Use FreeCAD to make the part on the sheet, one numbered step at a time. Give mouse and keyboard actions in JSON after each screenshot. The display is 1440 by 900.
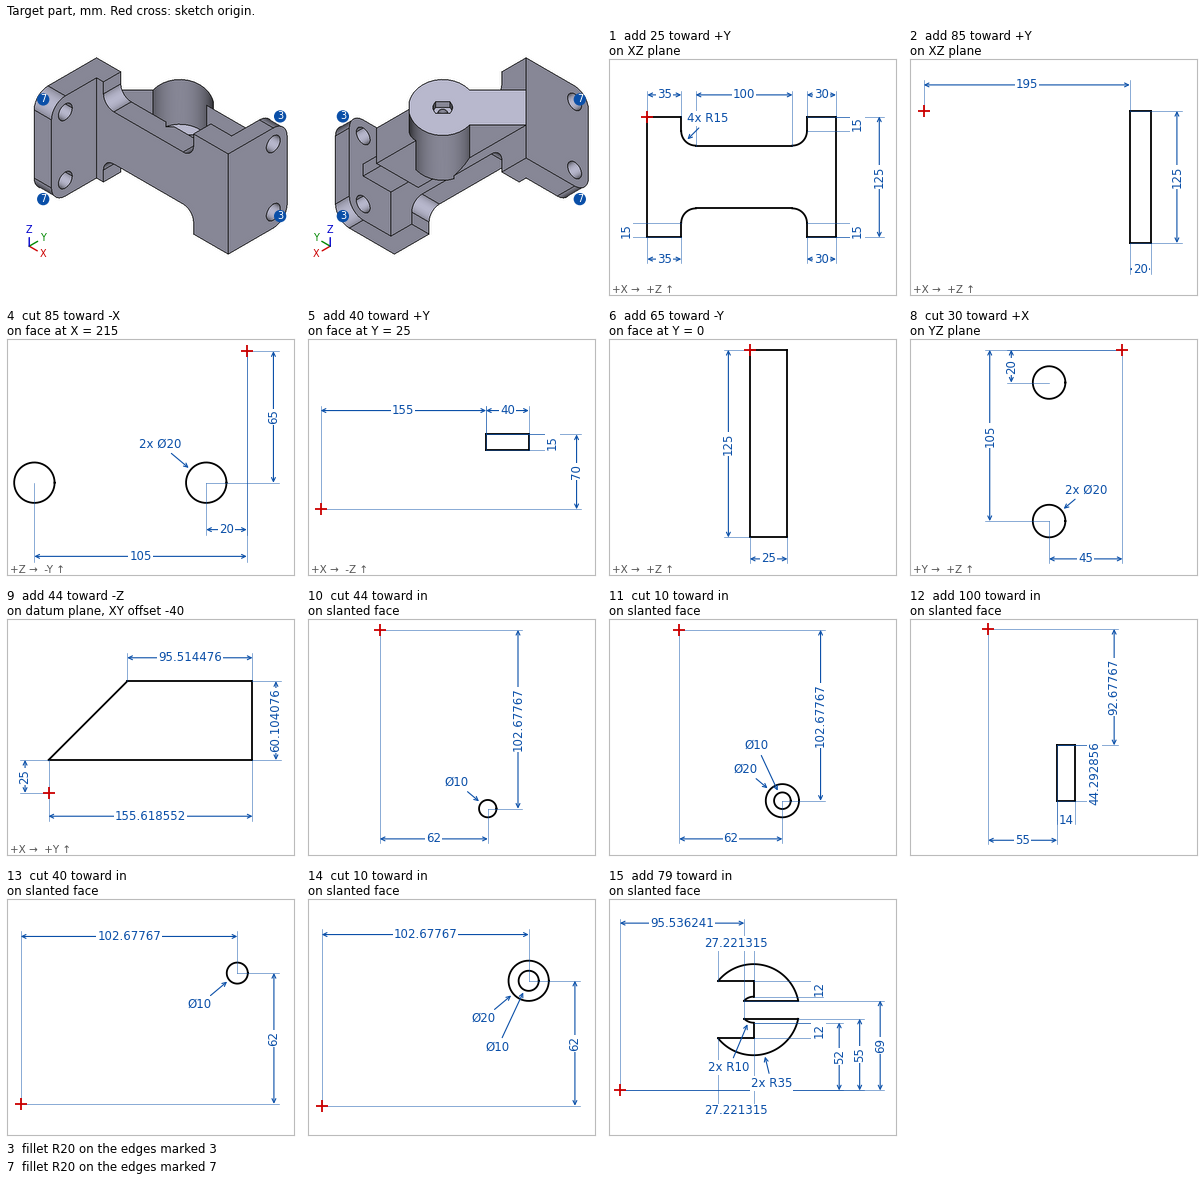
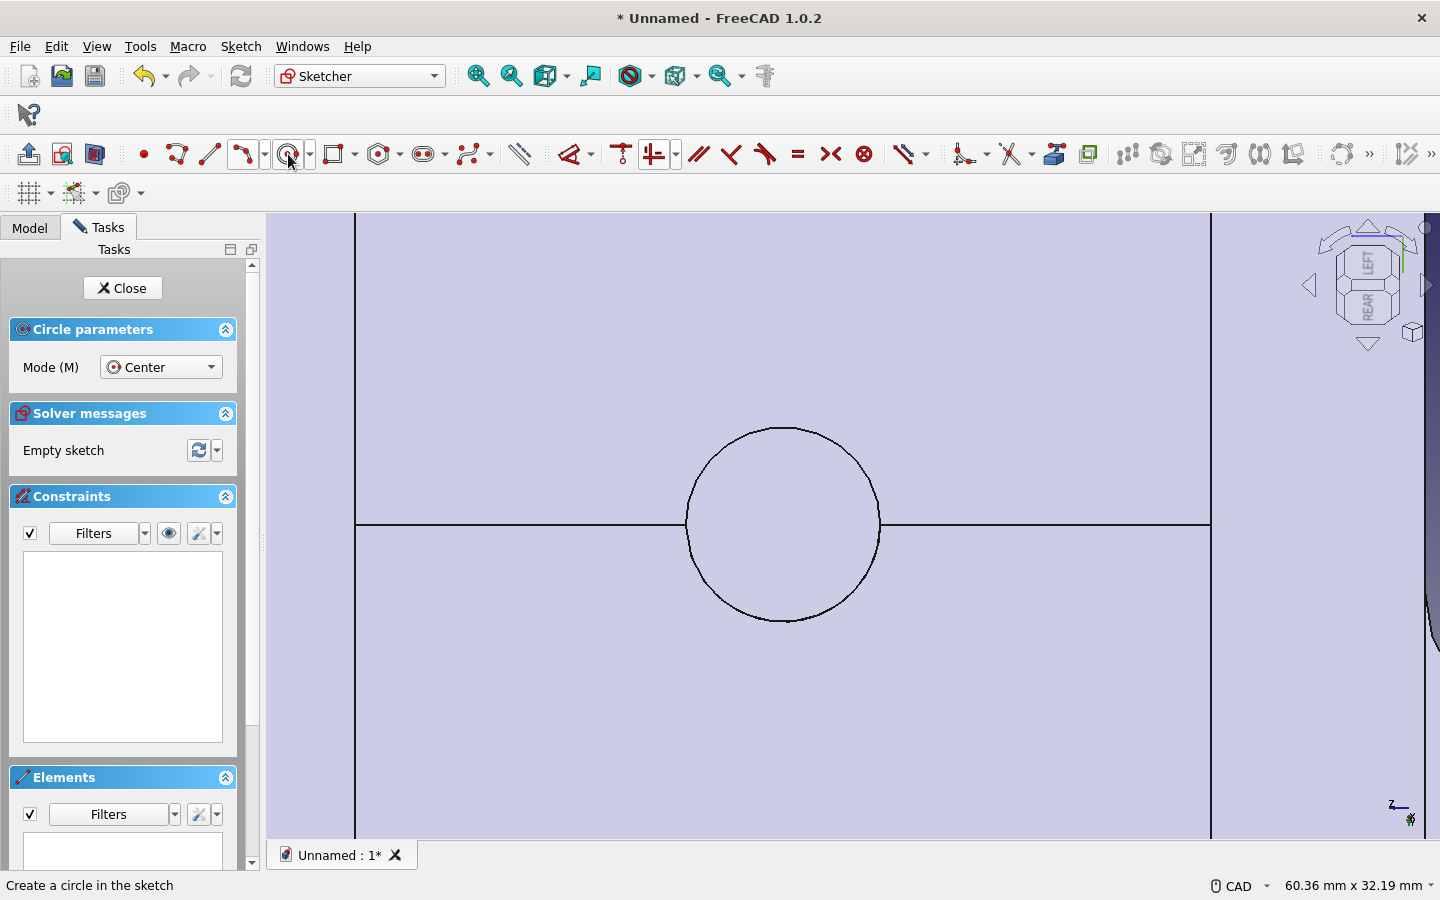
{"action": "left_click", "coordinate": [783, 525]}
{"action": "left_click", "coordinate": [921, 387]}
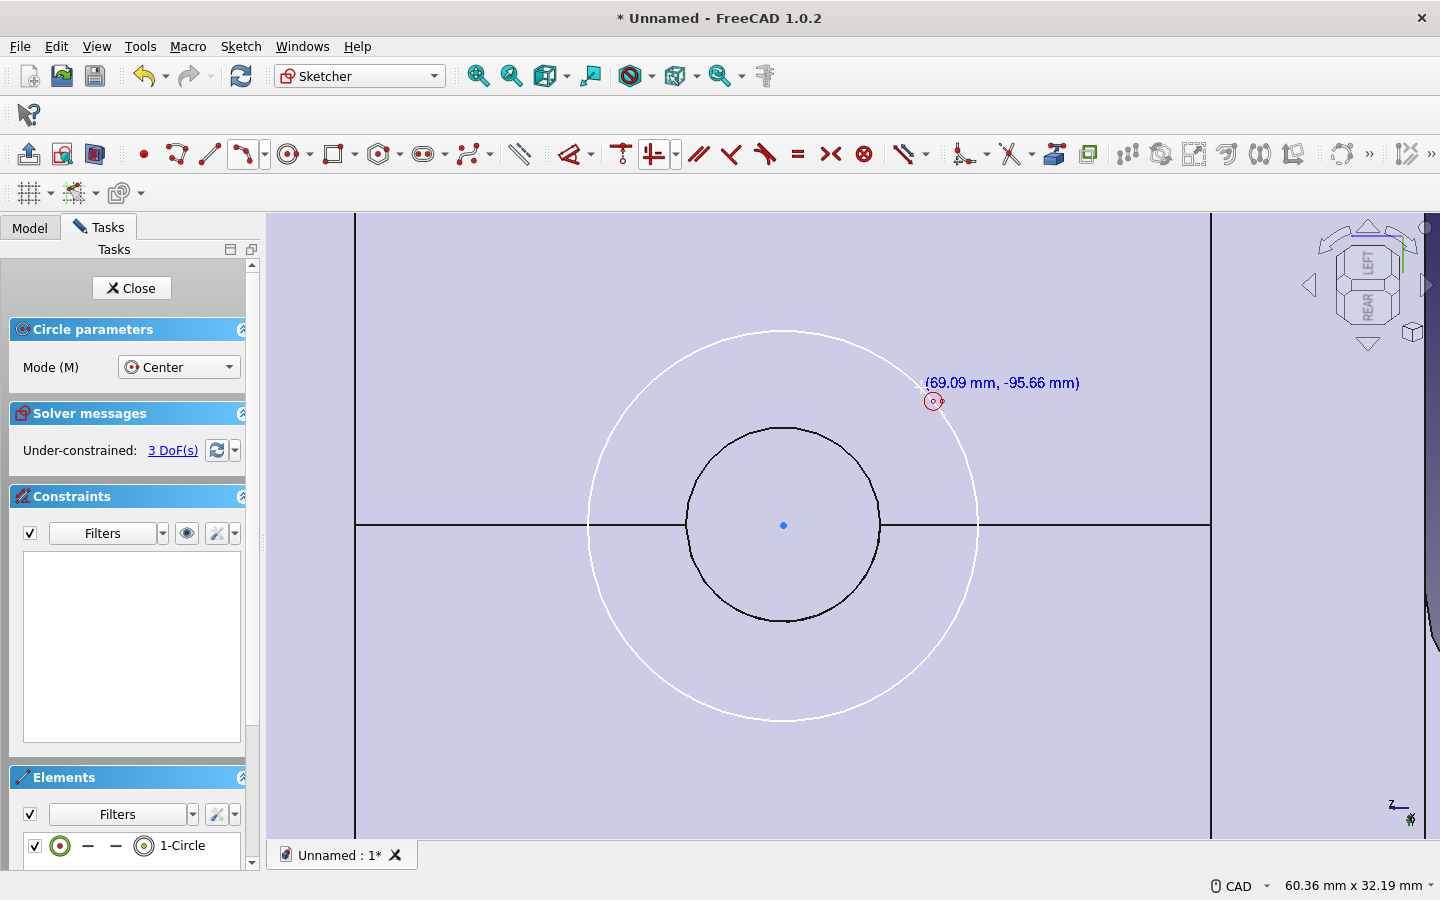
{"action": "left_click", "coordinate": [783, 526]}
{"action": "left_click", "coordinate": [852, 456]}
{"action": "key", "text": "Escape"}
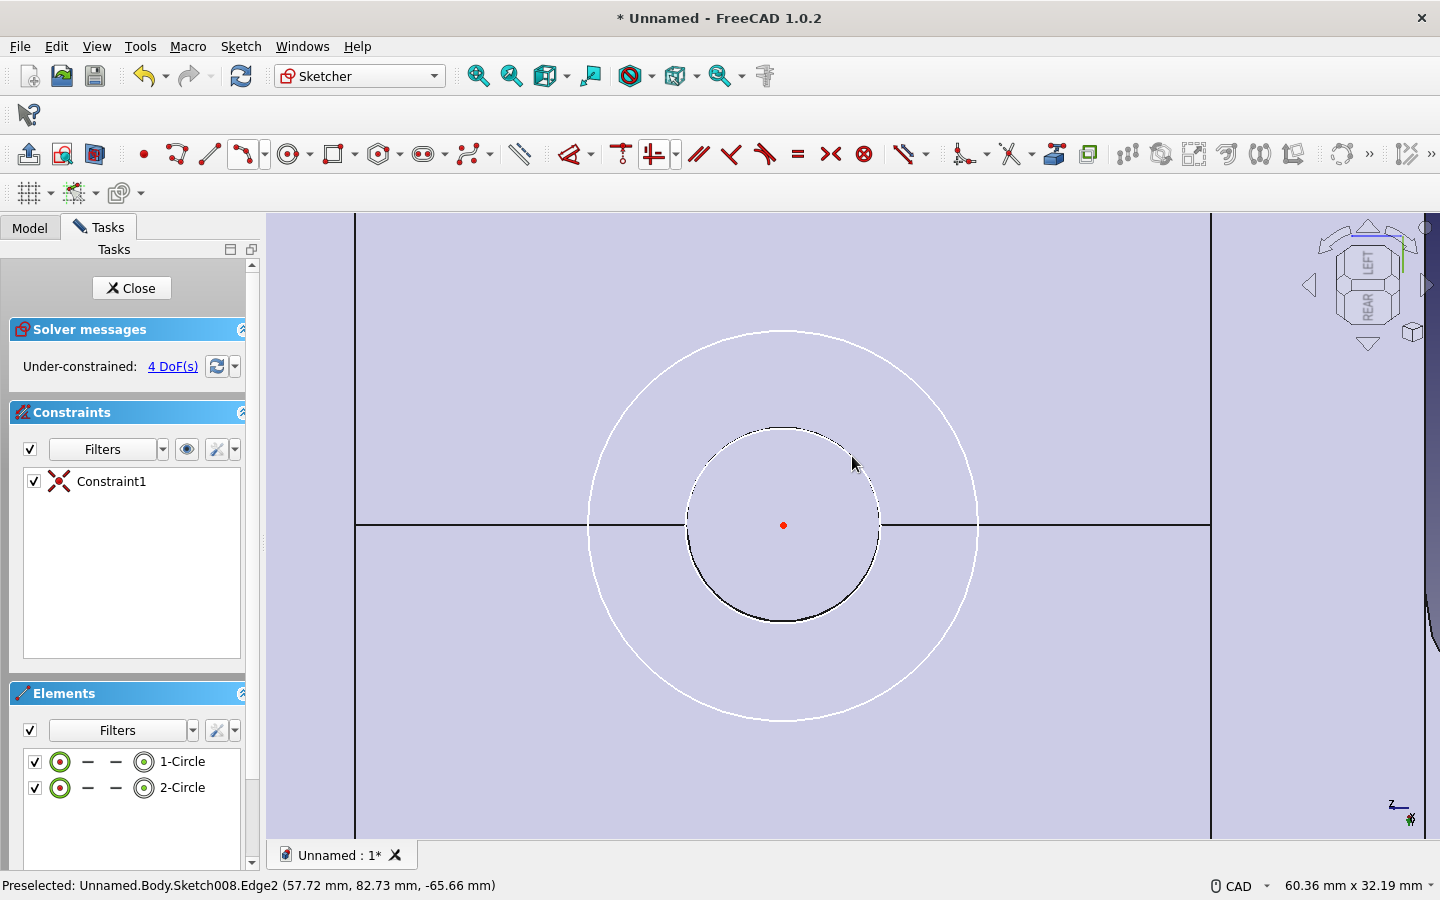
{"action": "left_click", "coordinate": [568, 154]}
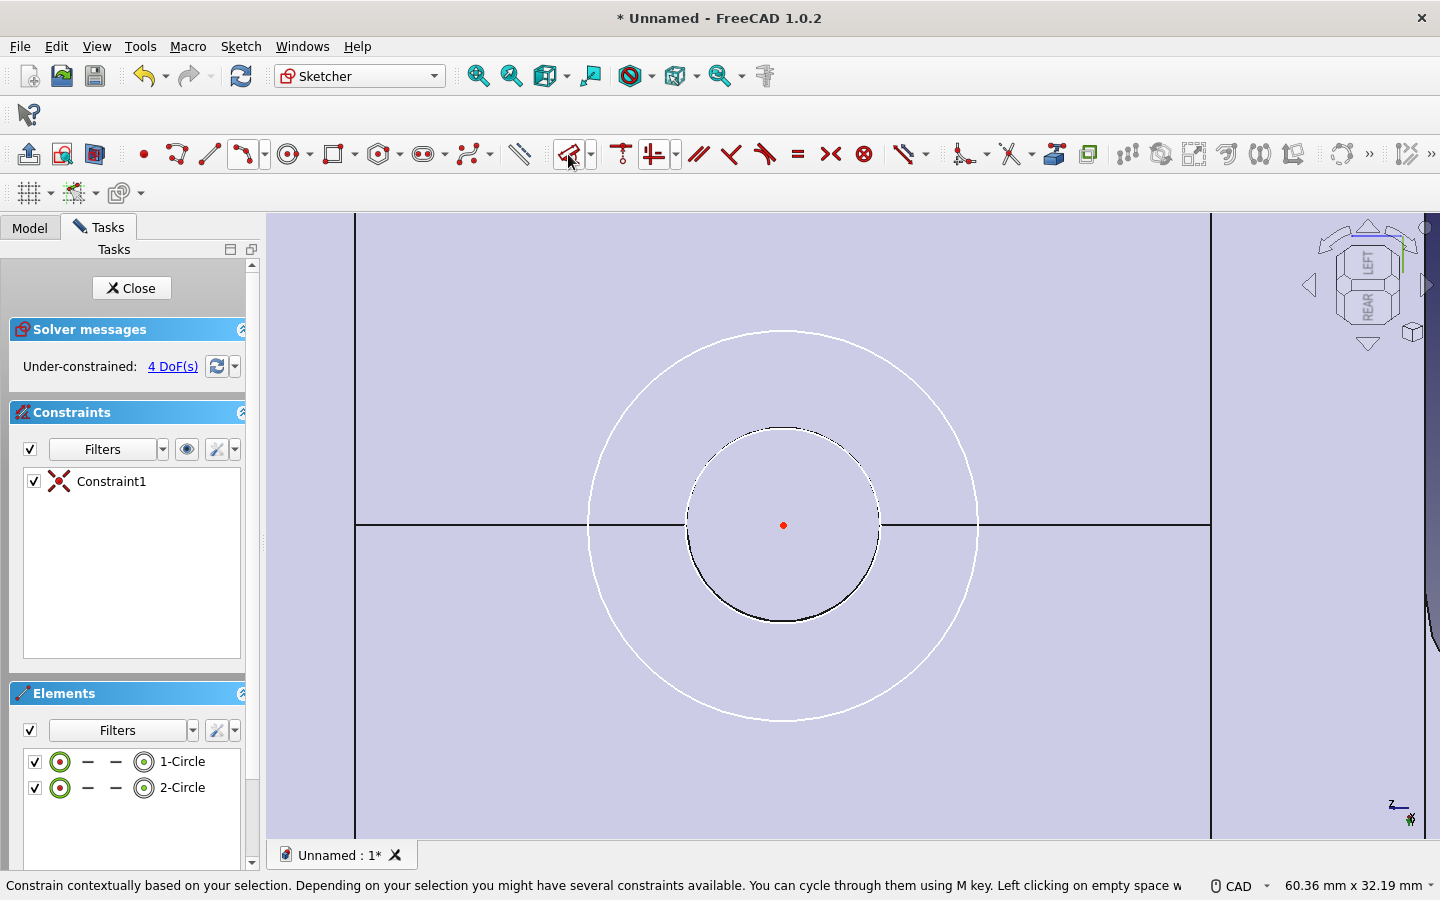
{"action": "left_click", "coordinate": [921, 388]}
{"action": "left_click", "coordinate": [944, 365]}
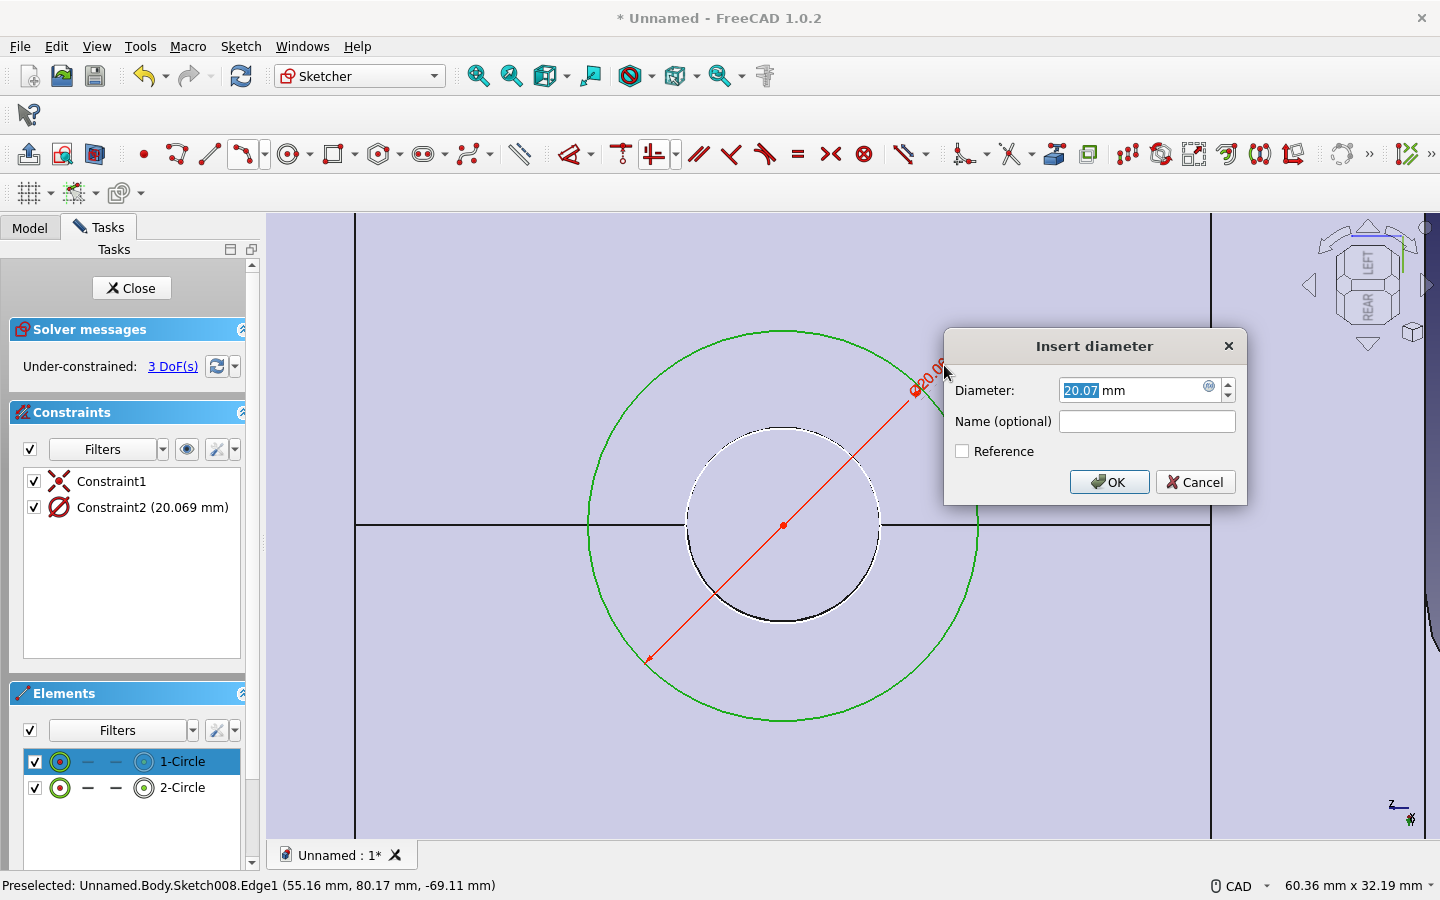
{"action": "type", "text": "20"}
{"action": "key", "text": "Return"}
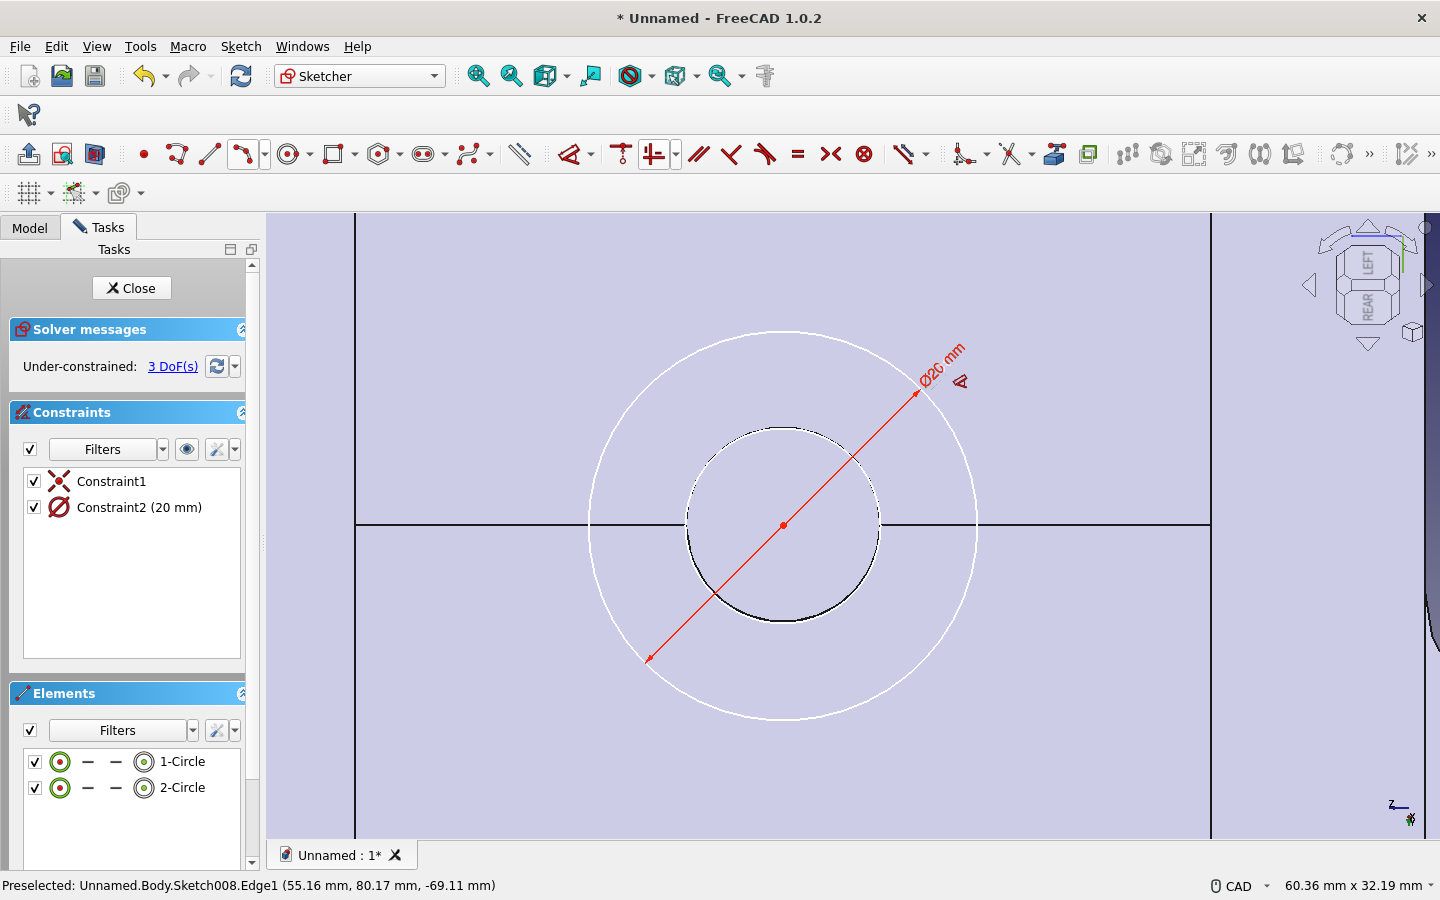
{"action": "left_click", "coordinate": [852, 457]}
{"action": "left_click", "coordinate": [875, 434]}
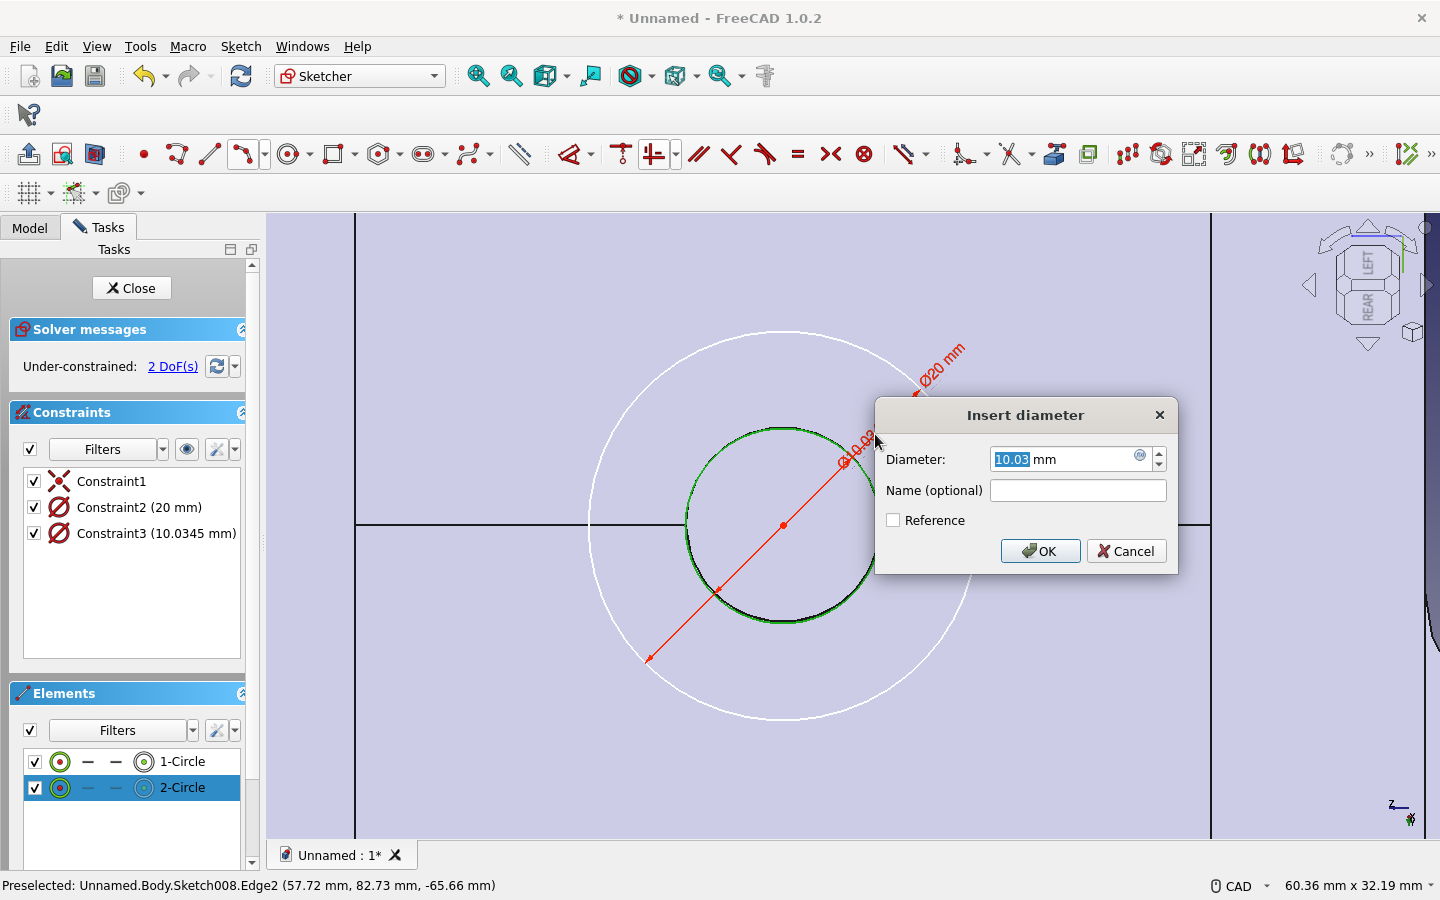
{"action": "type", "text": "10"}
{"action": "key", "text": "Return"}